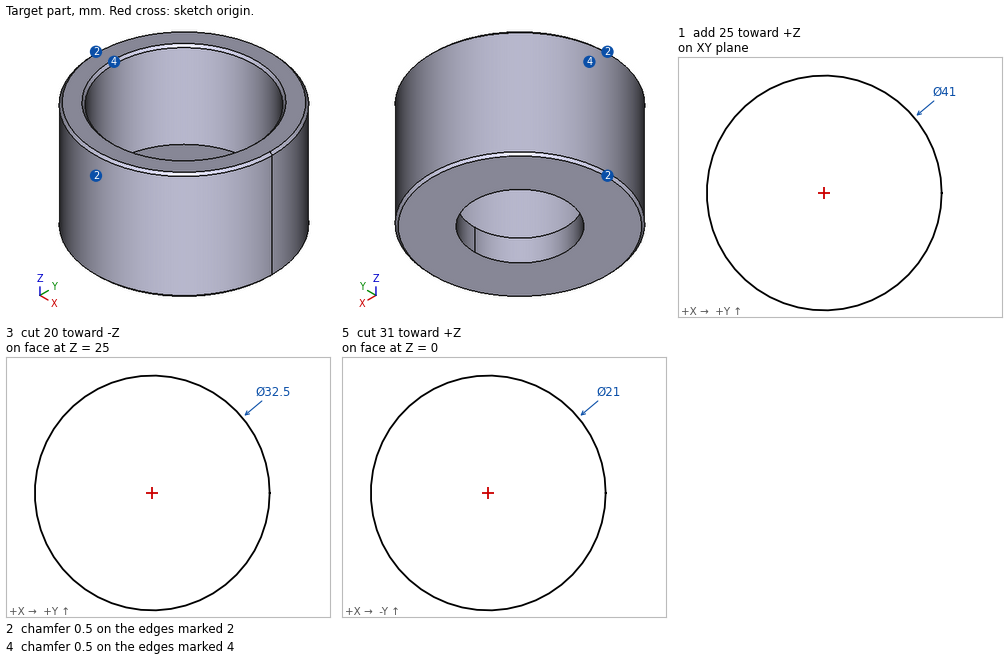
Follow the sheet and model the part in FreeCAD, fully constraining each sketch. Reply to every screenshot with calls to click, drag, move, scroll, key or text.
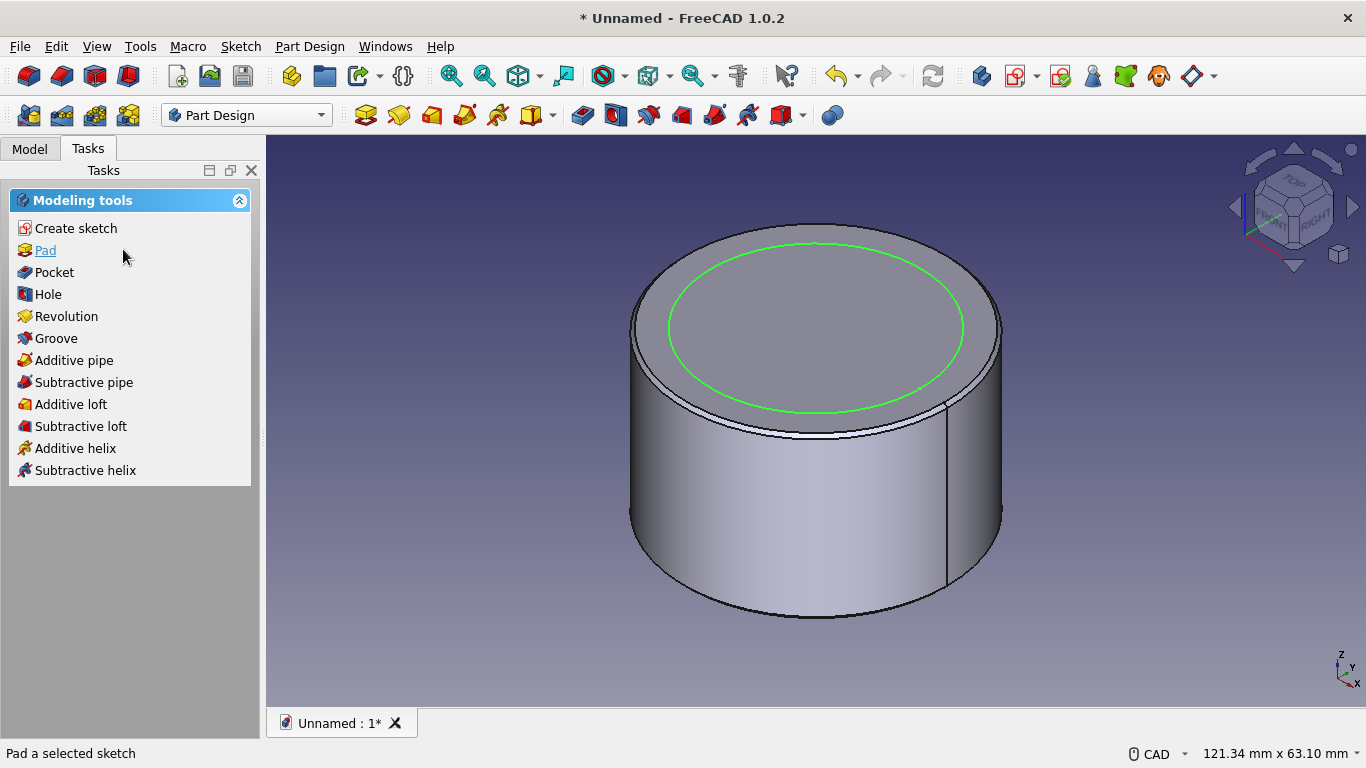
click(583, 116)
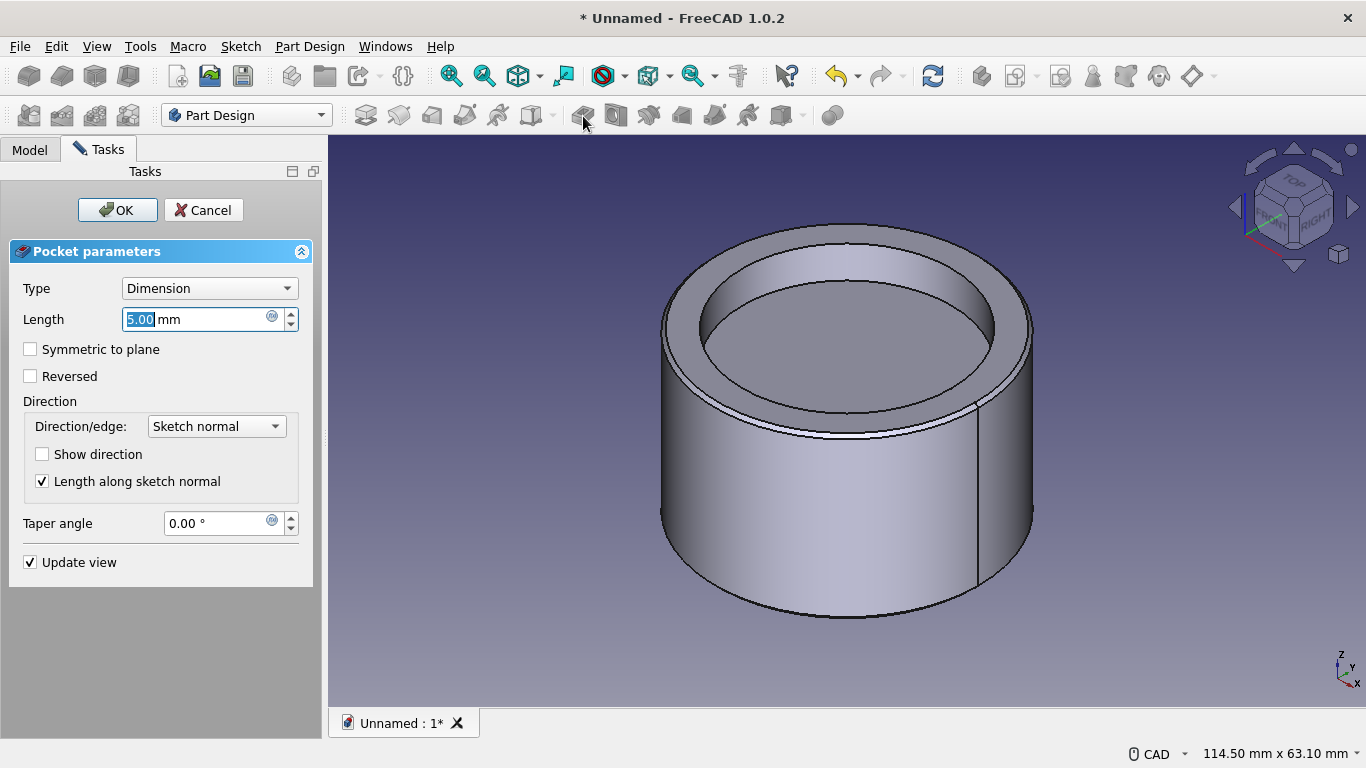
text(20)
key(Tab)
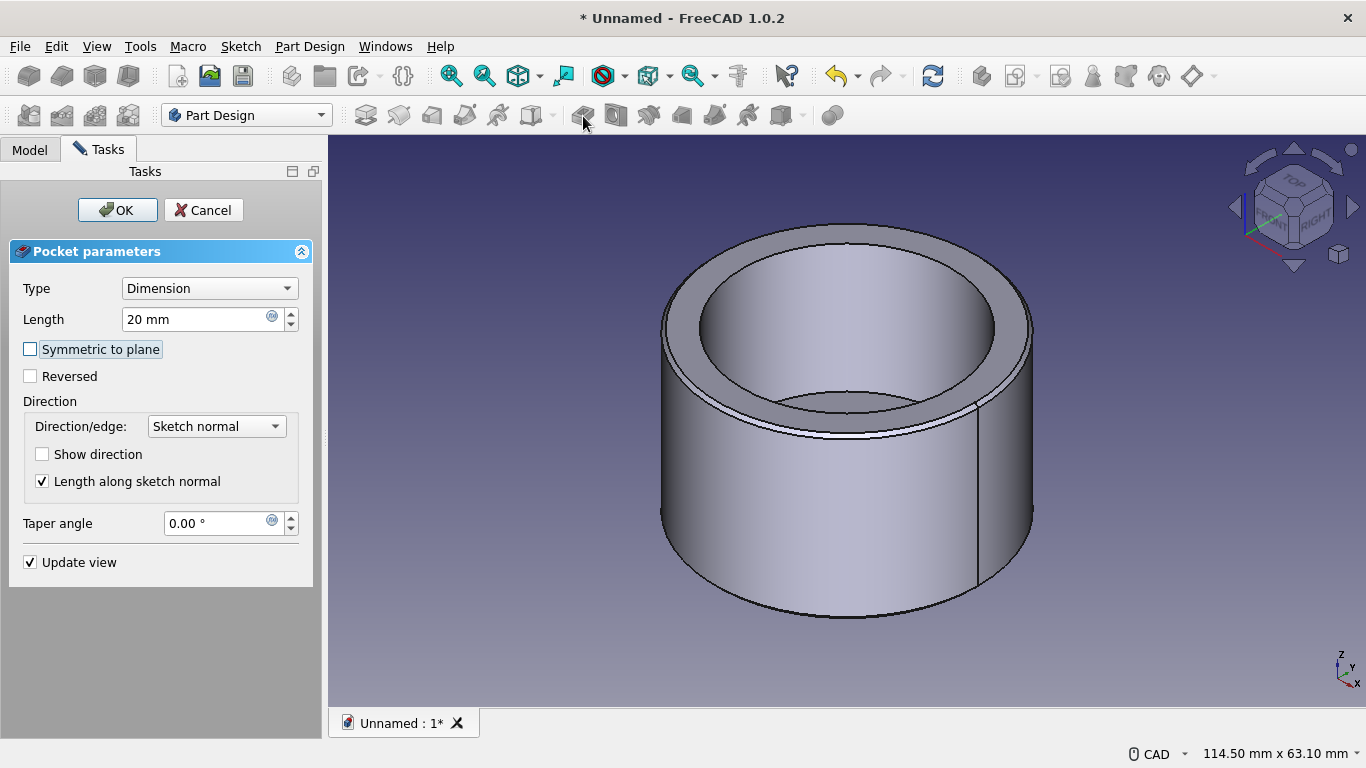
click(118, 210)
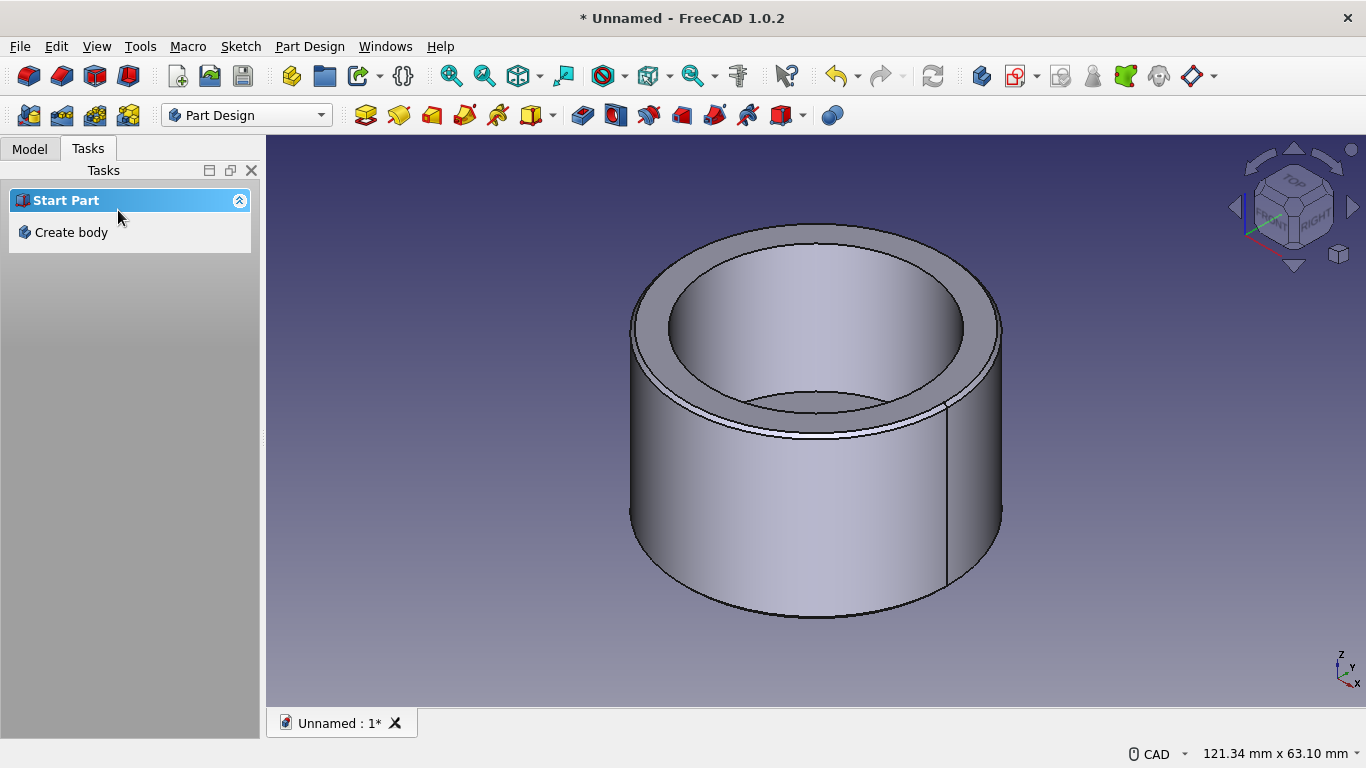
click(712, 267)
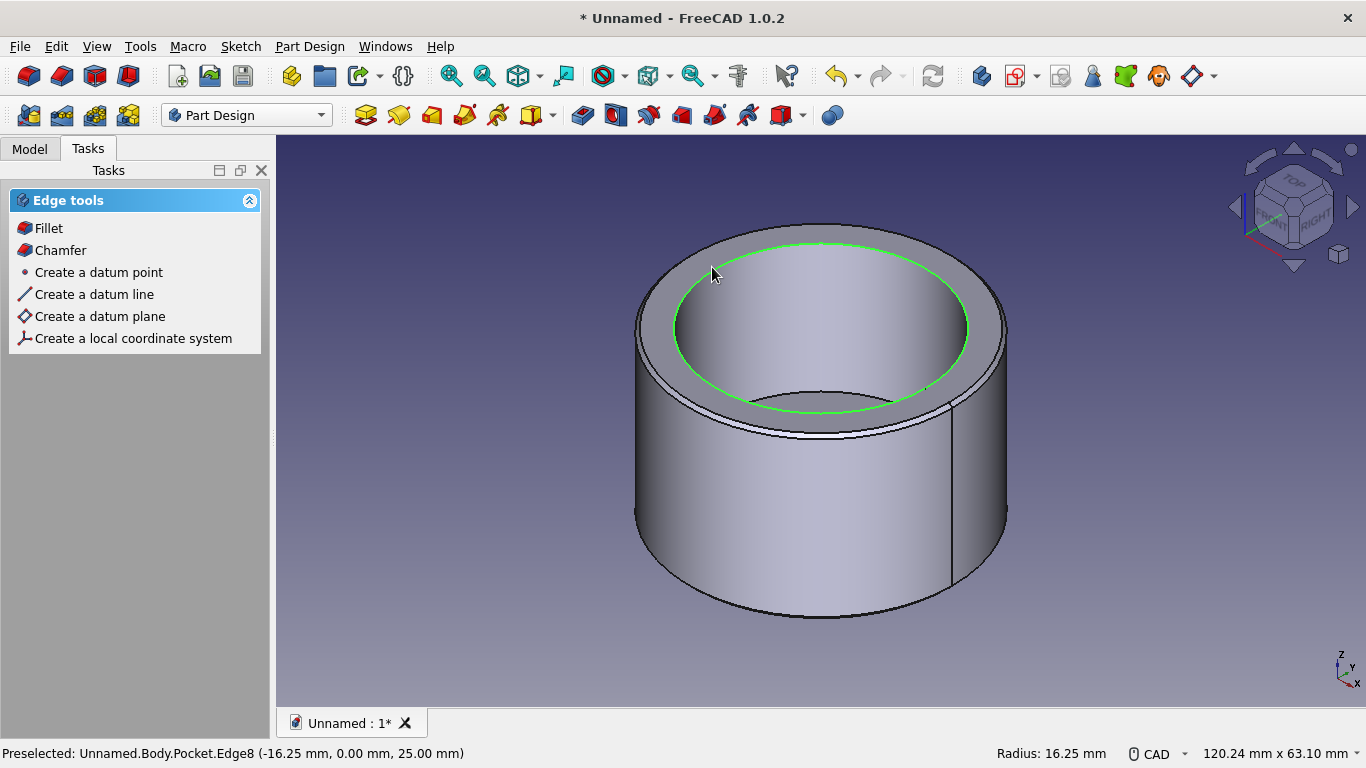
click(62, 76)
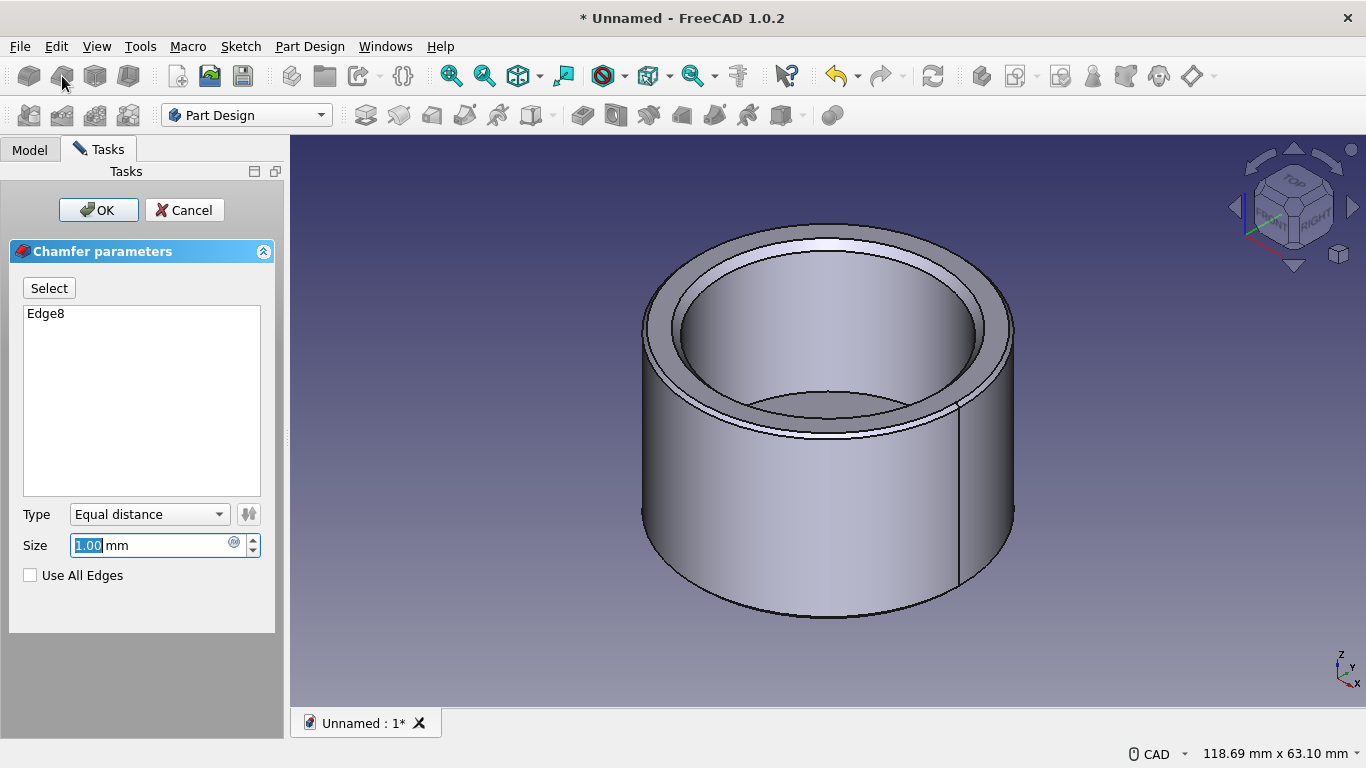
text(0.5)
key(Tab)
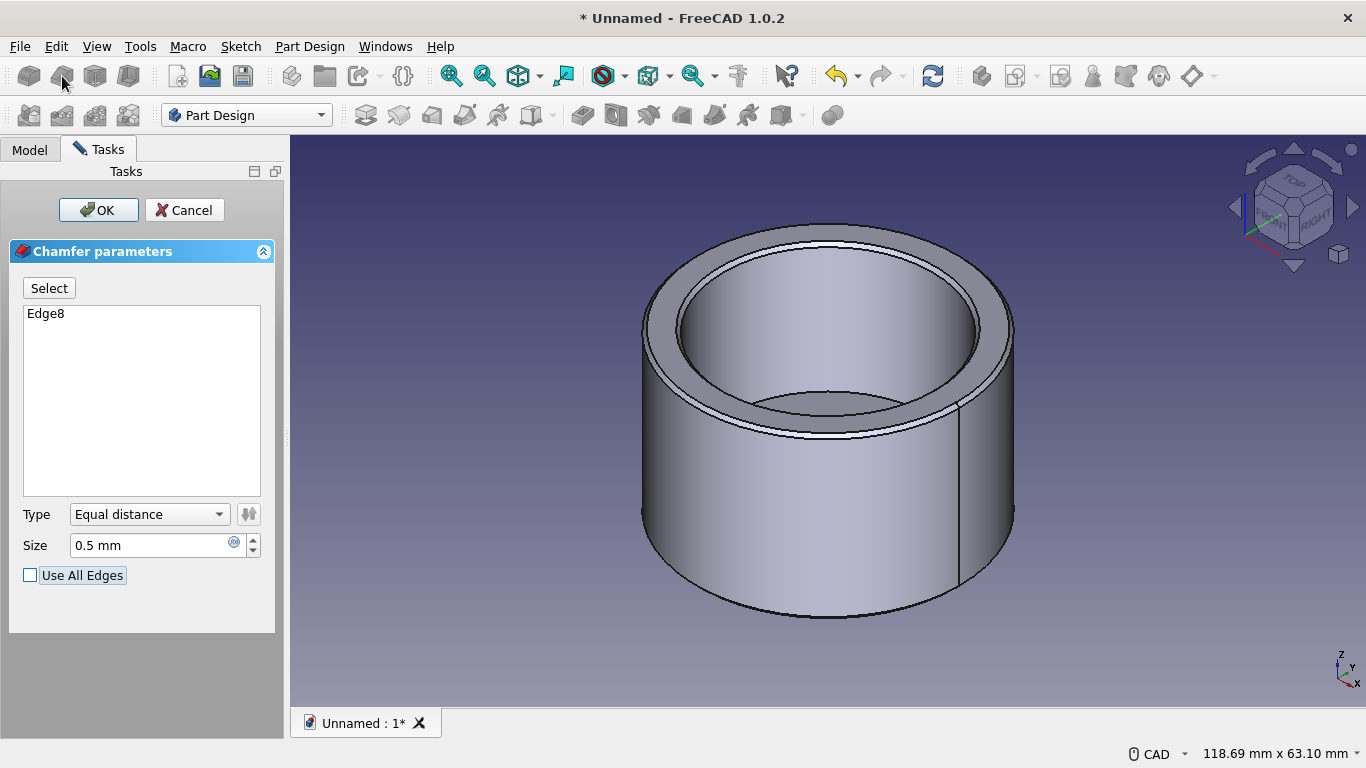
click(99, 210)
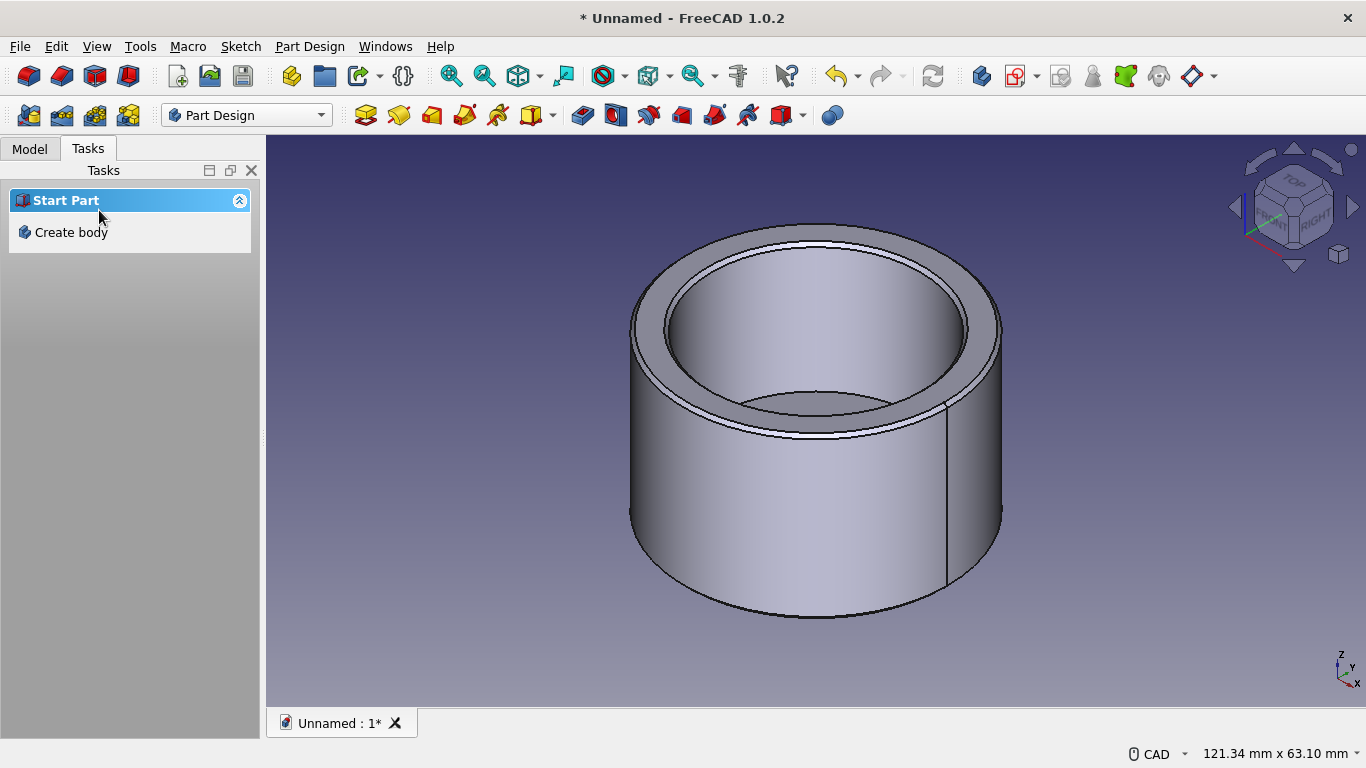
key(5)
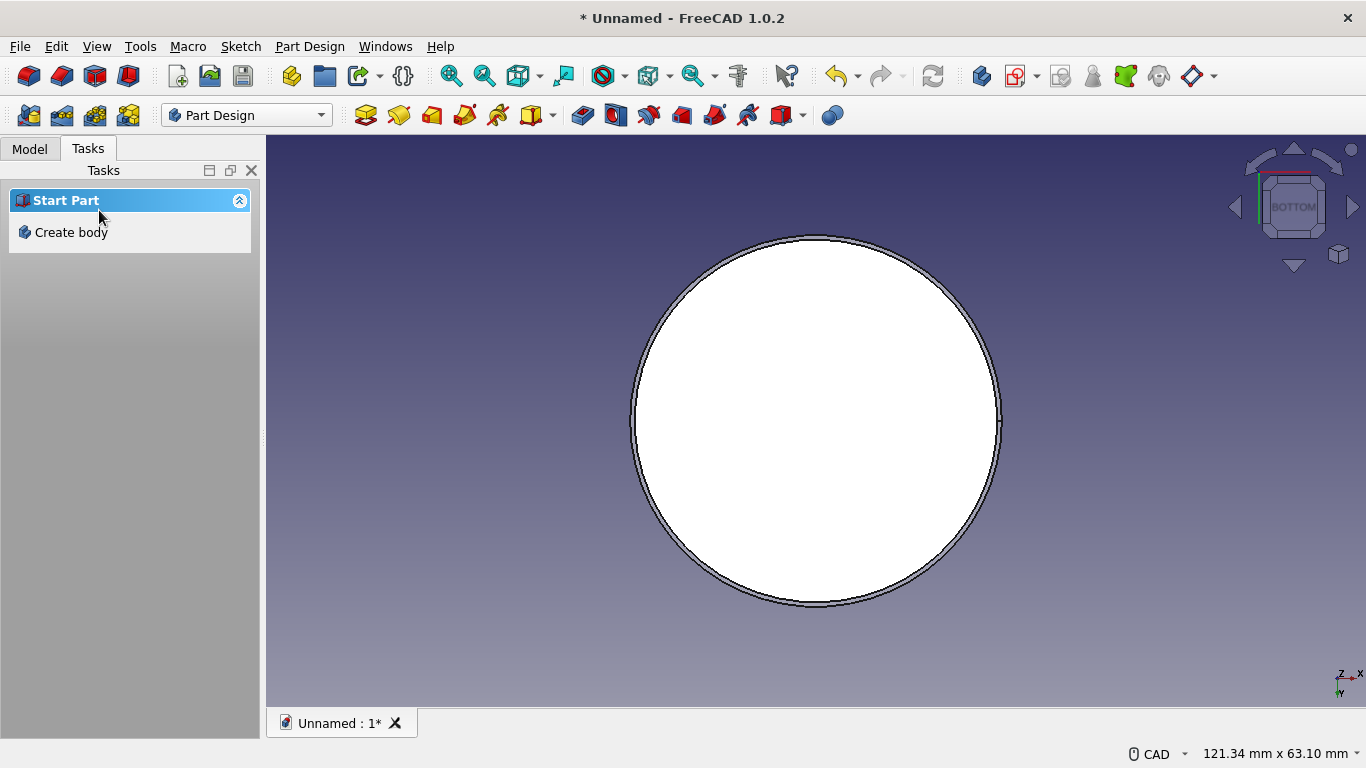
click(816, 420)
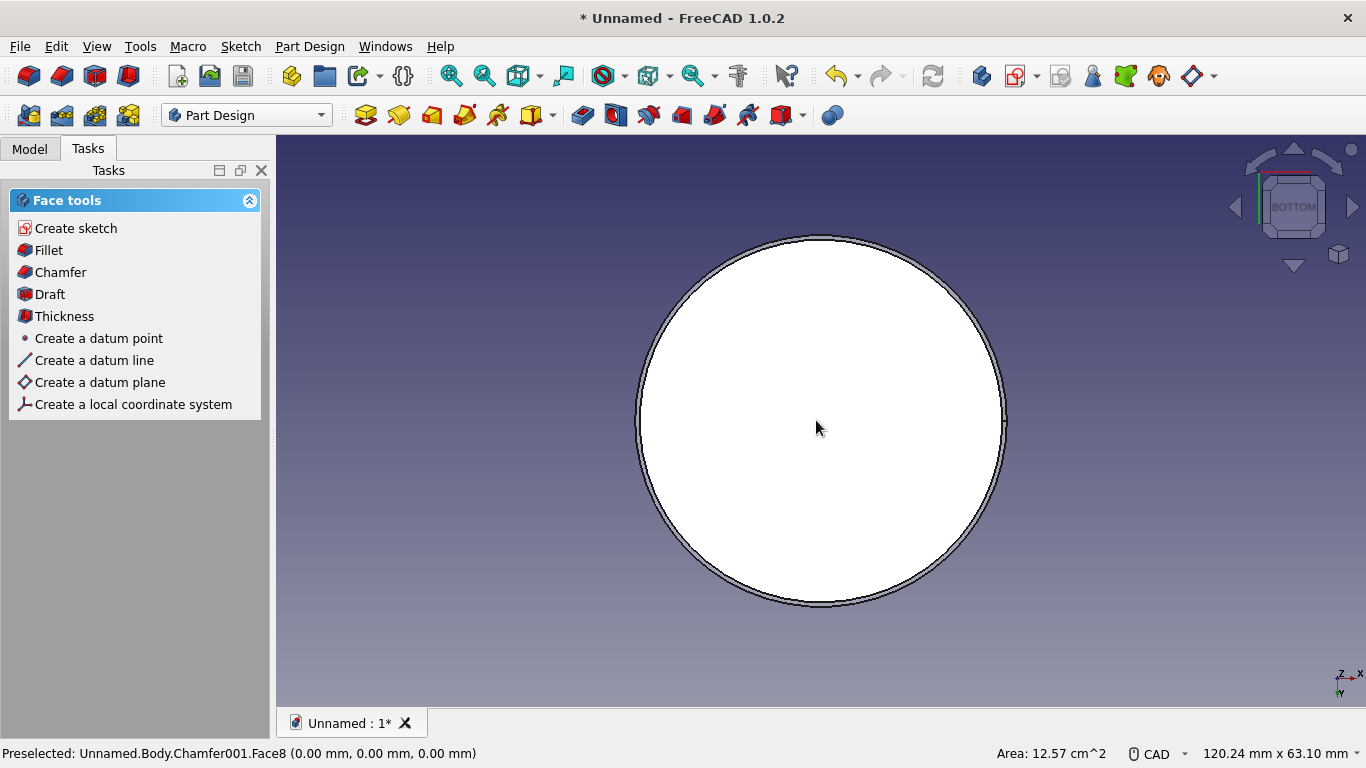
click(1014, 76)